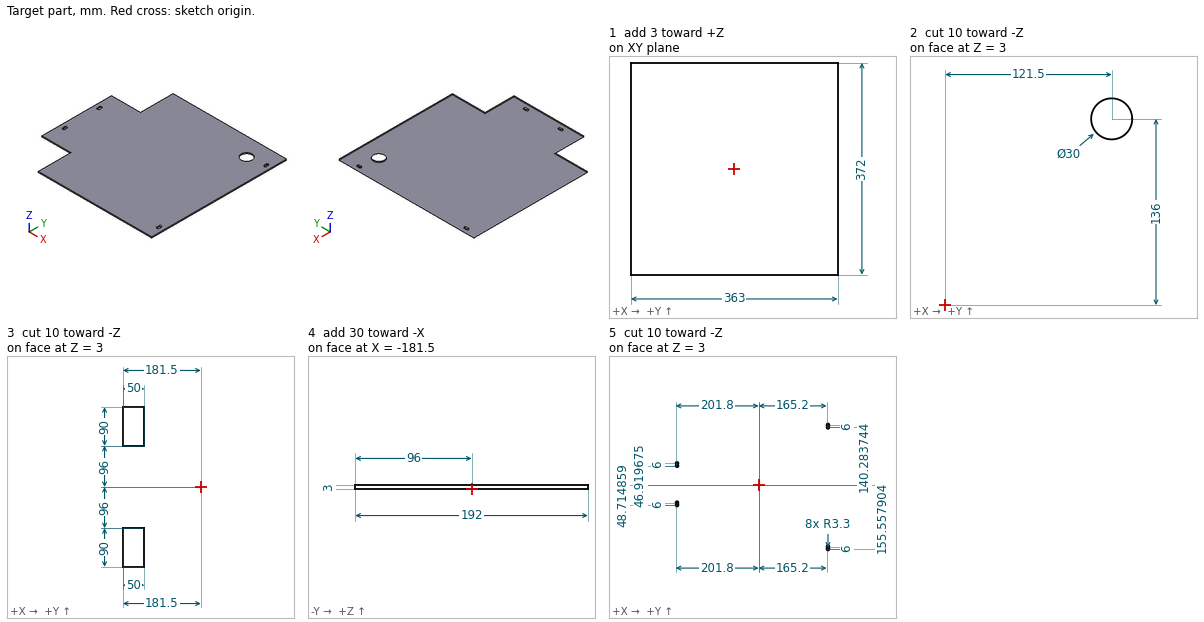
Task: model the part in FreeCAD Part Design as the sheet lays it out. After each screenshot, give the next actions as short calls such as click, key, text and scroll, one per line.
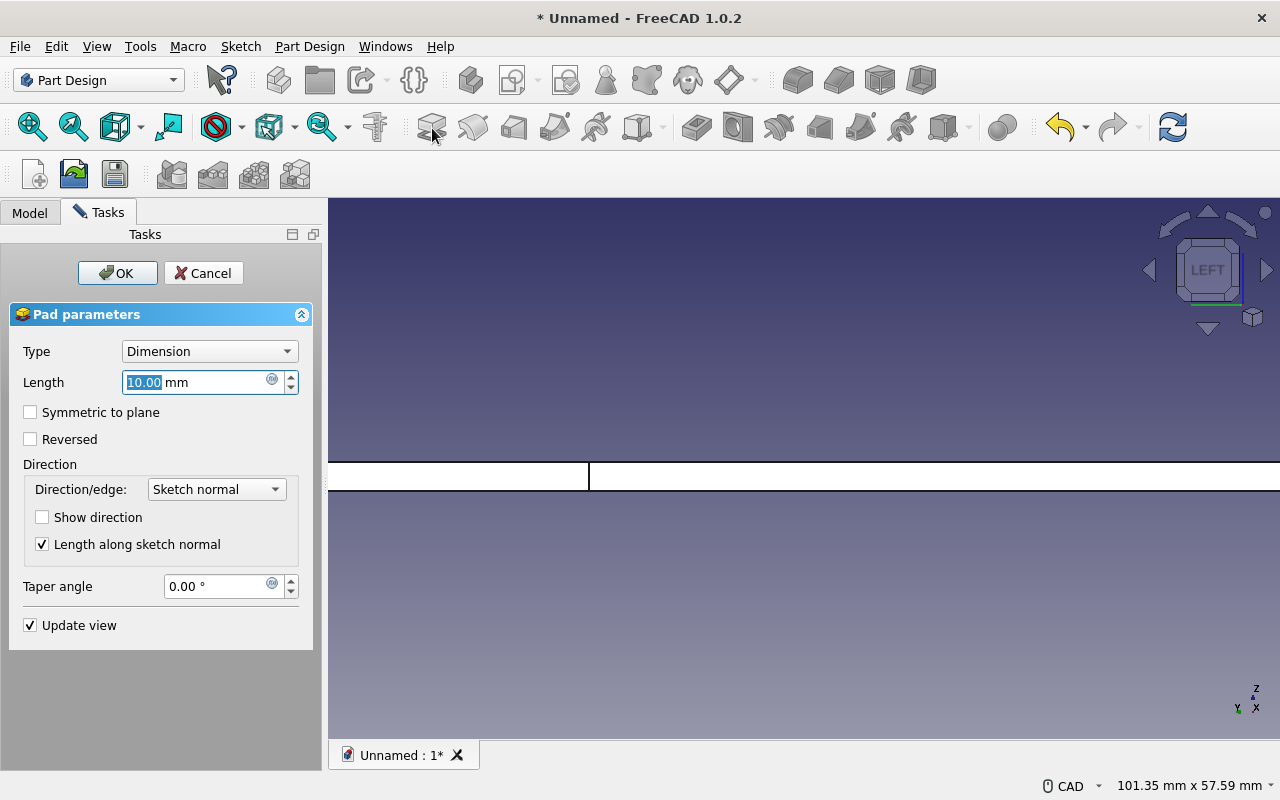
text(30)
key(Tab)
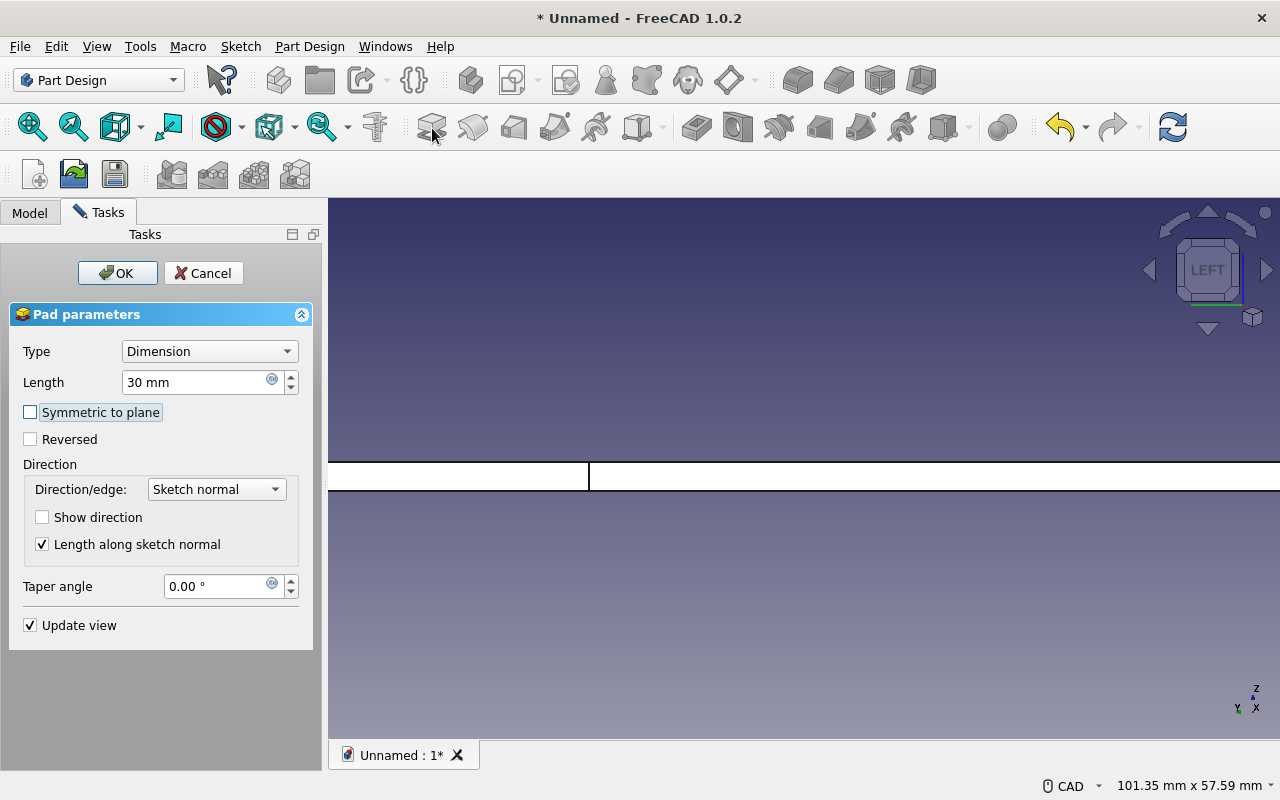
click(118, 273)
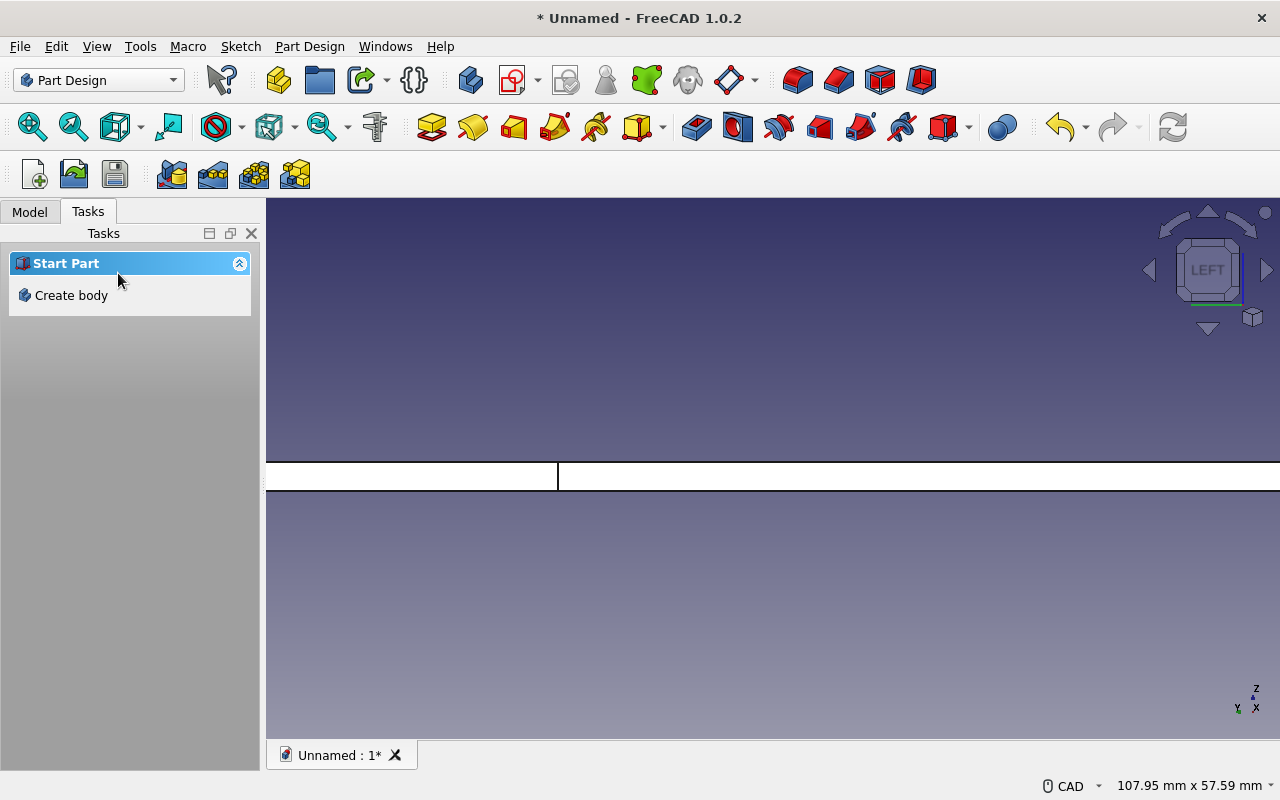
click(33, 128)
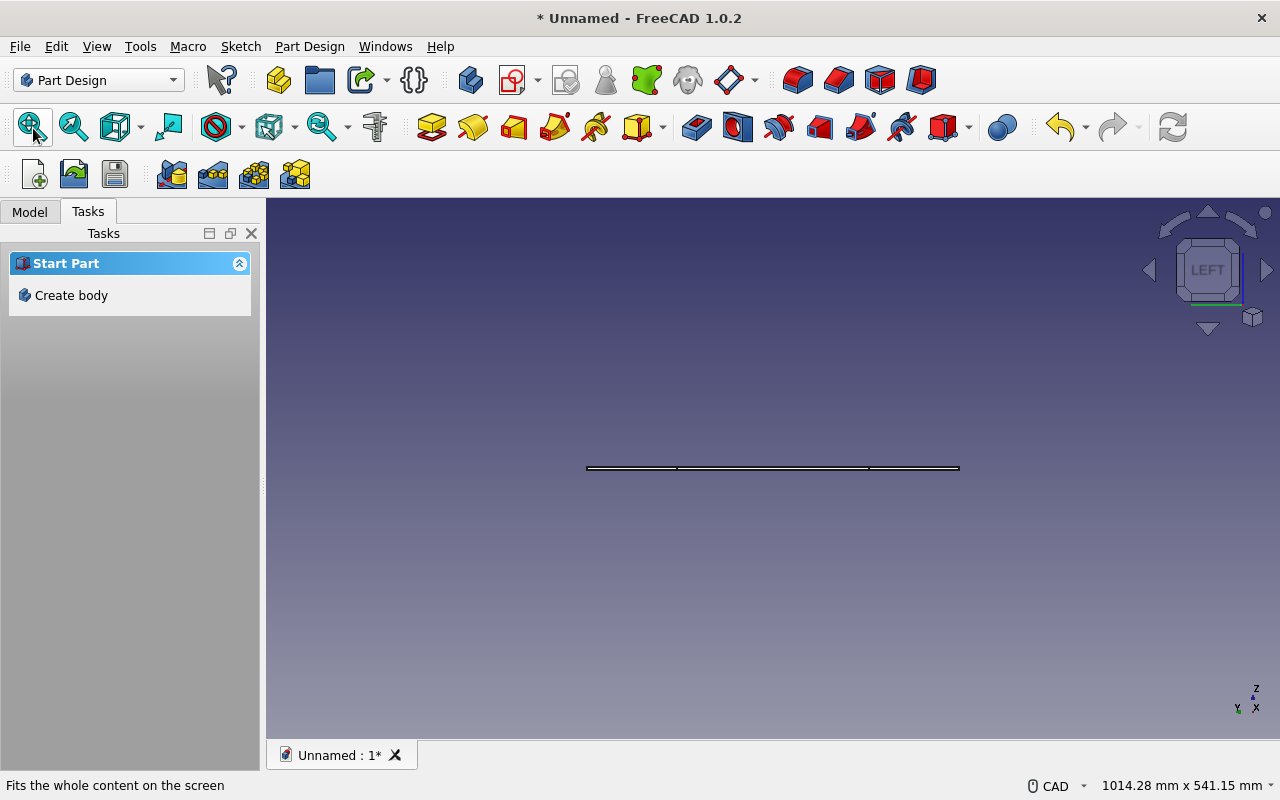
key(0)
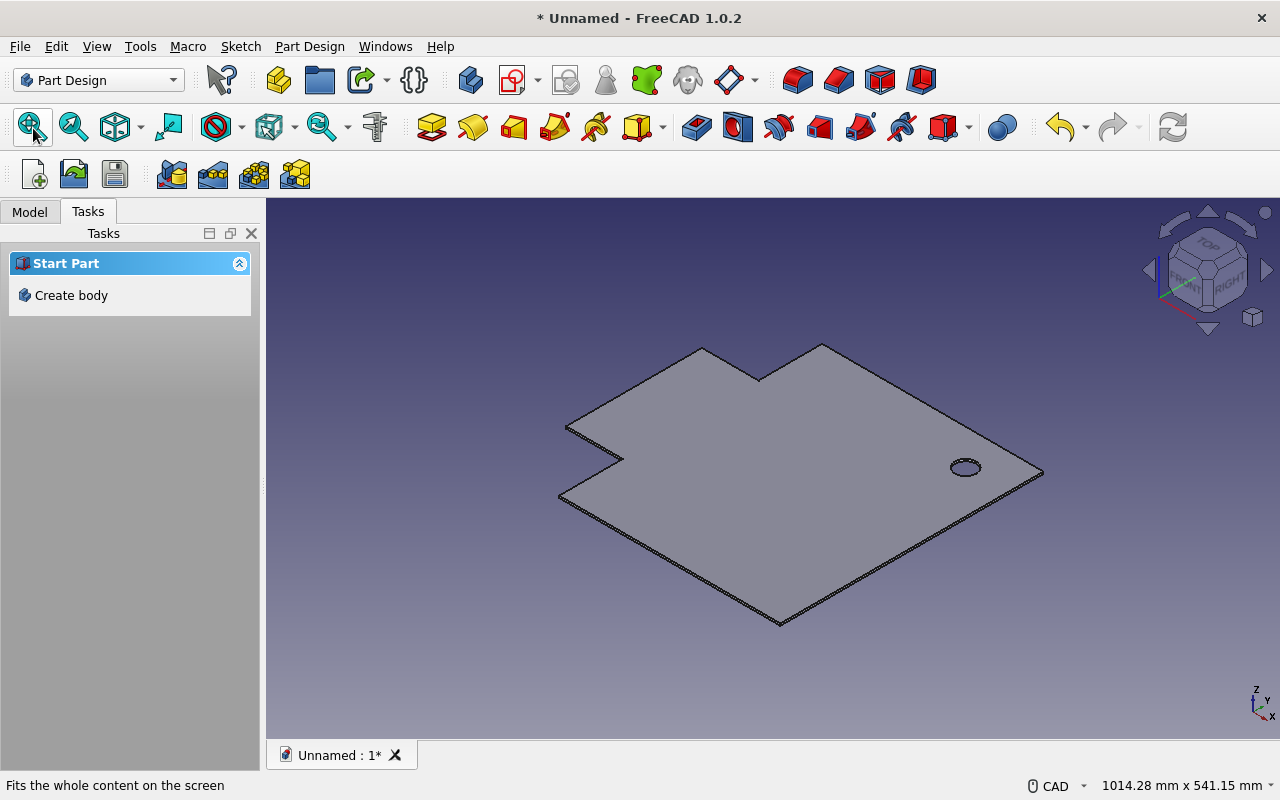
click(773, 466)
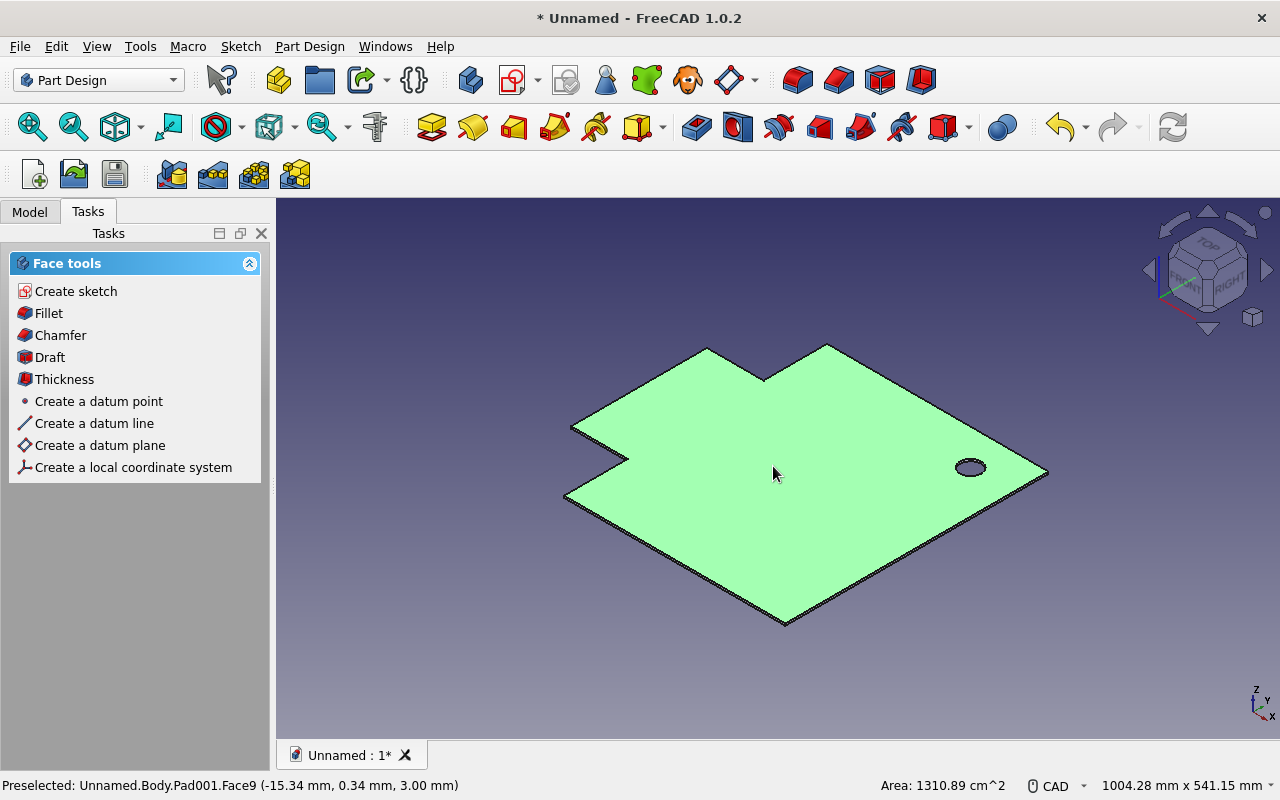
click(512, 80)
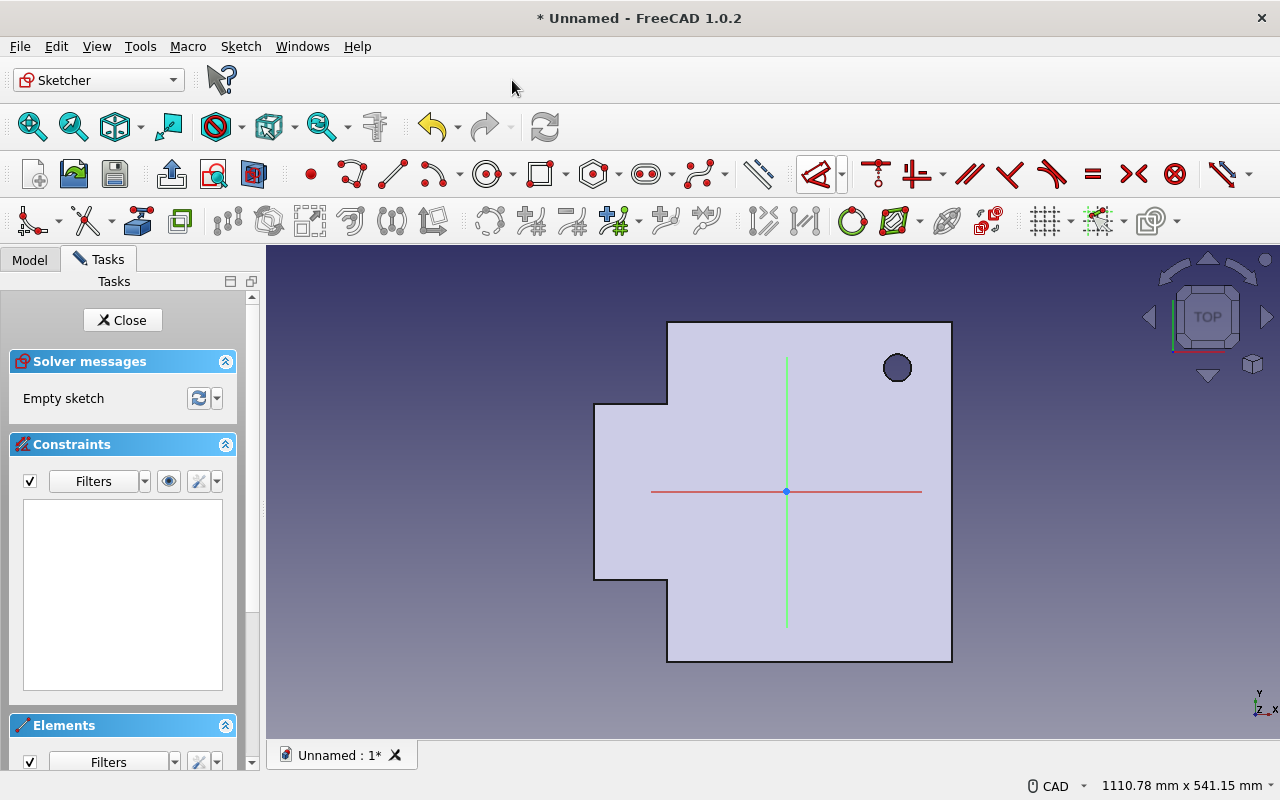
click(646, 174)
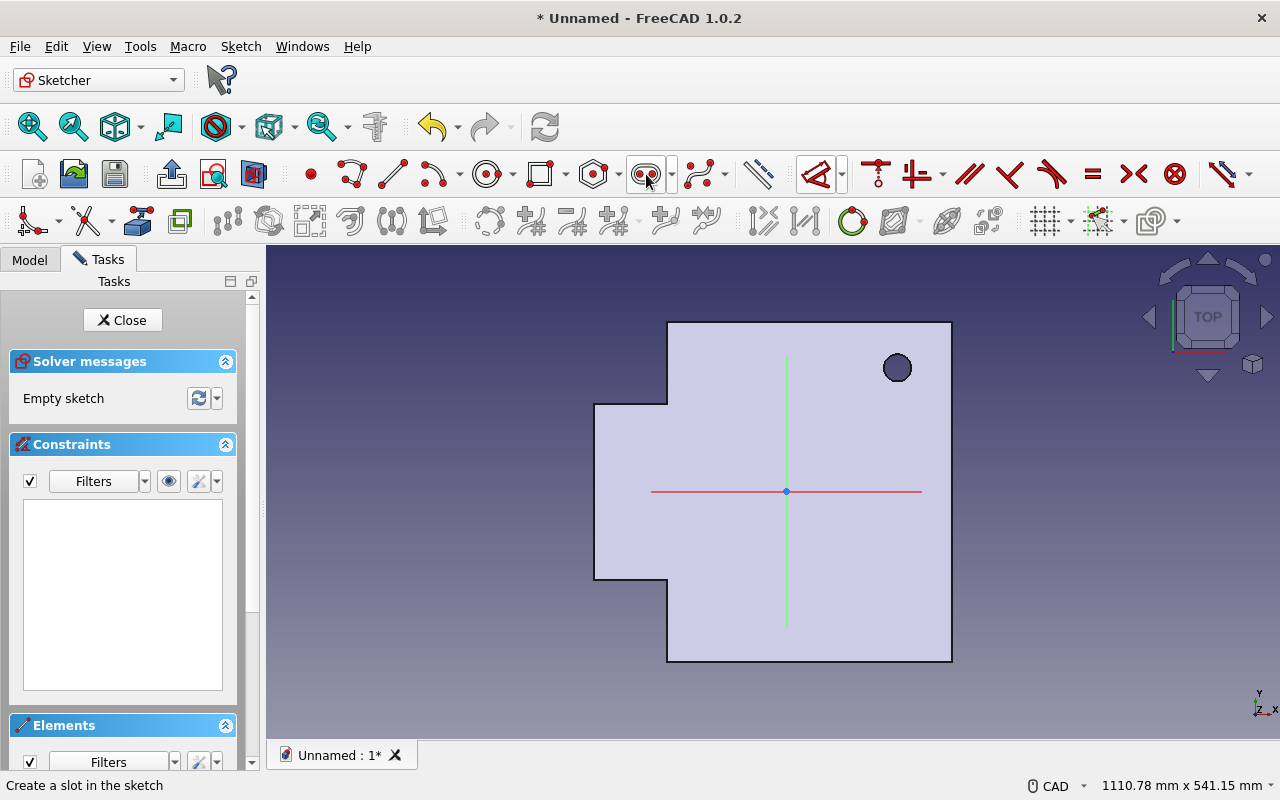
scroll(941, 634, up, 11)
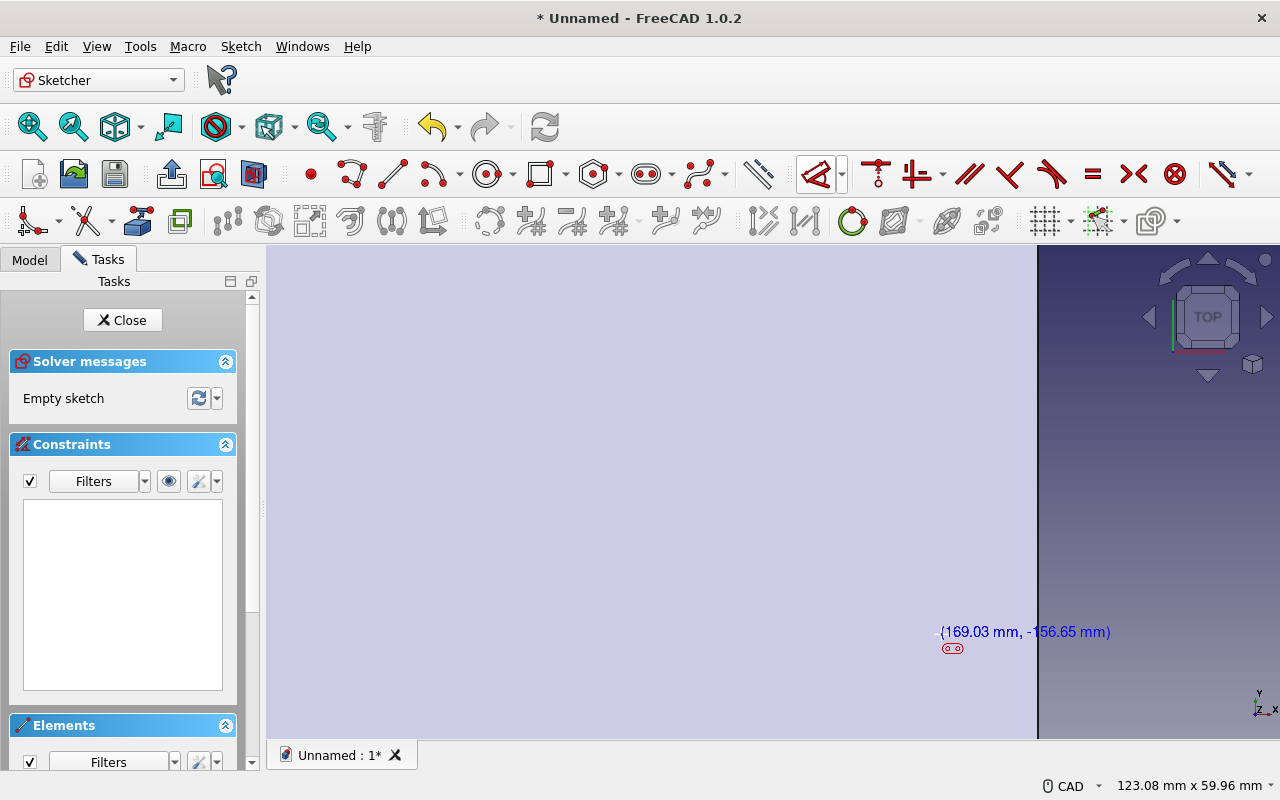
scroll(865, 630, down, 11)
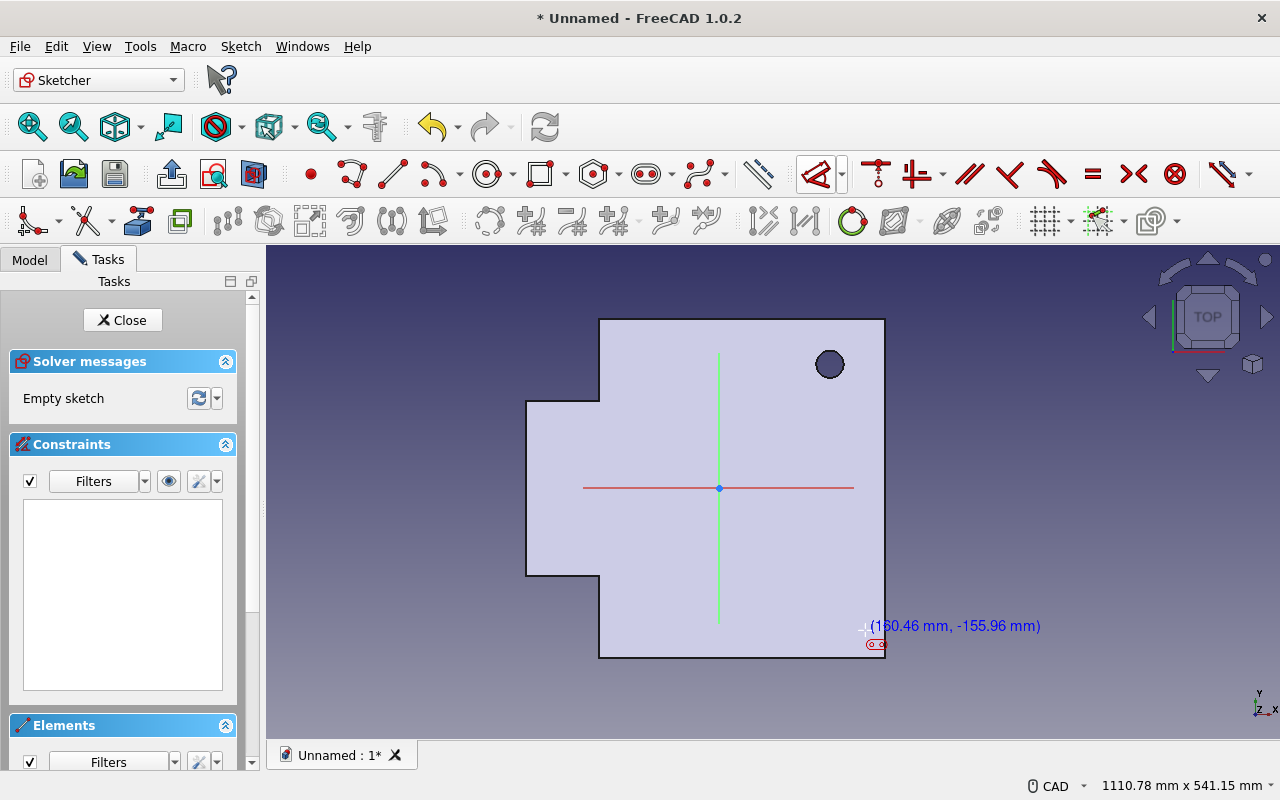
click(873, 630)